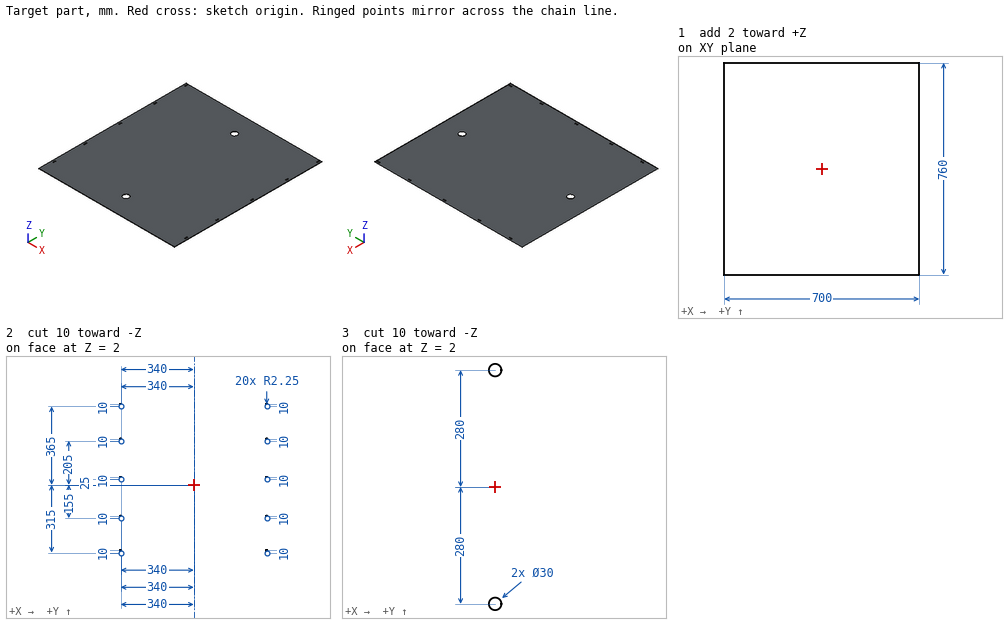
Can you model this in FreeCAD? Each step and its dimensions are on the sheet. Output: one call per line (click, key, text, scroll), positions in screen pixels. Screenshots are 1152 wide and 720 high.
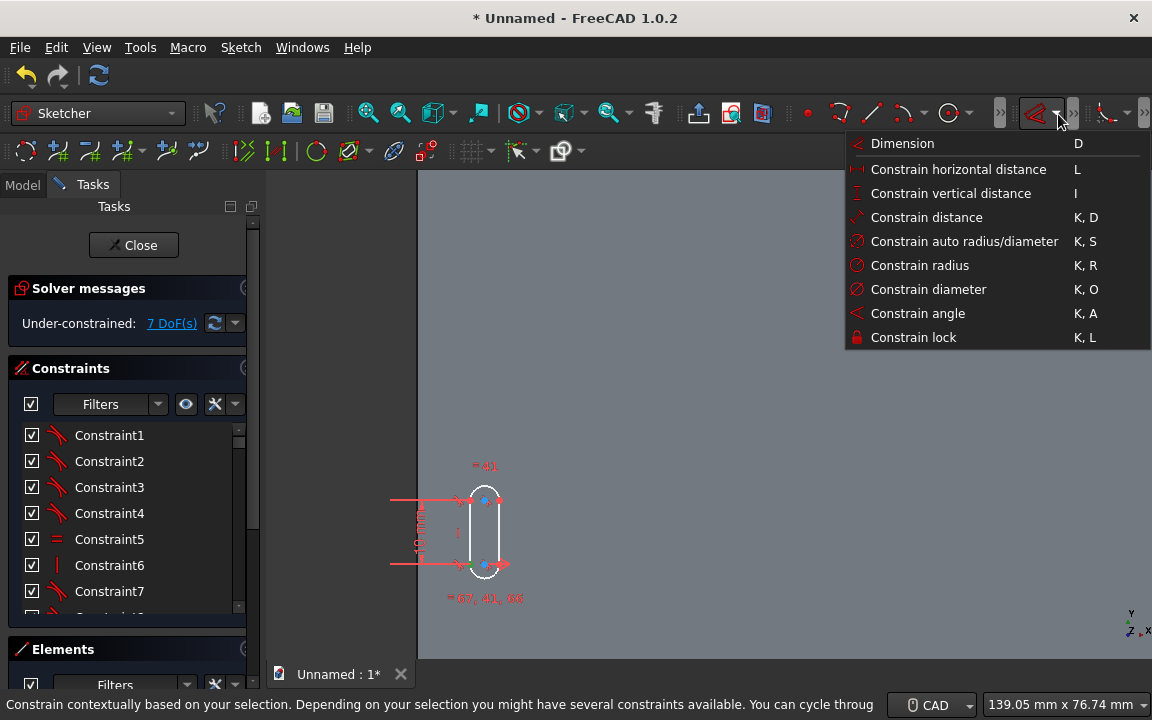
click(998, 193)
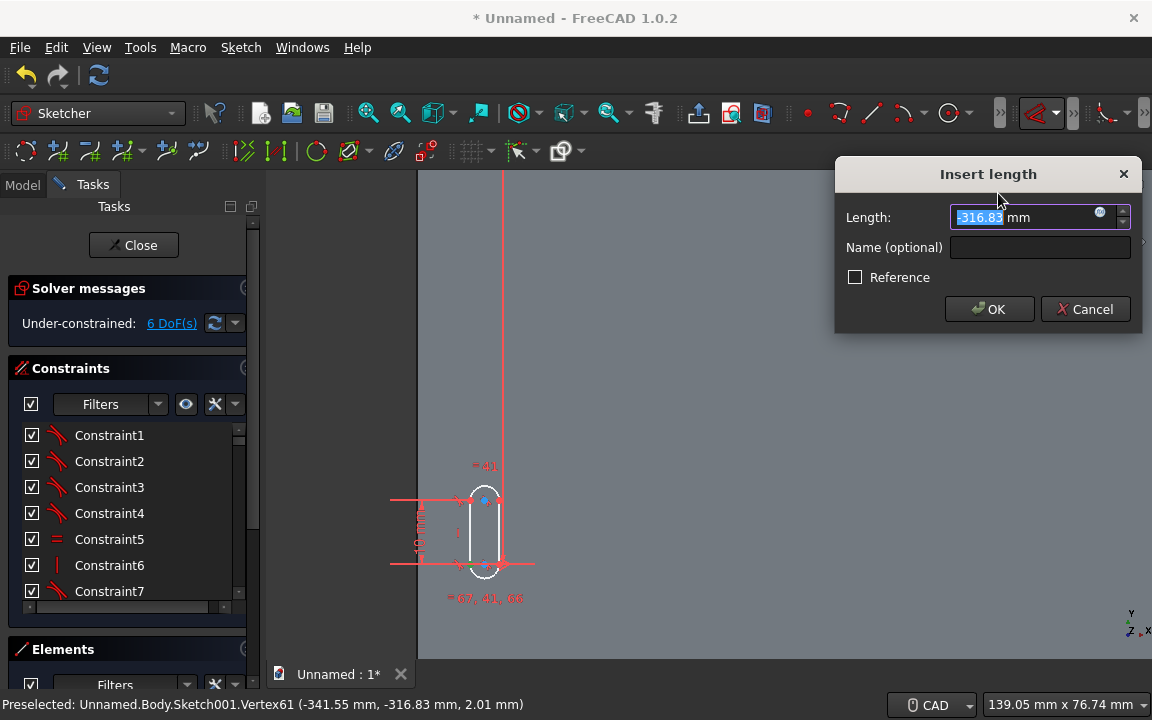
text(-315)
key(Return)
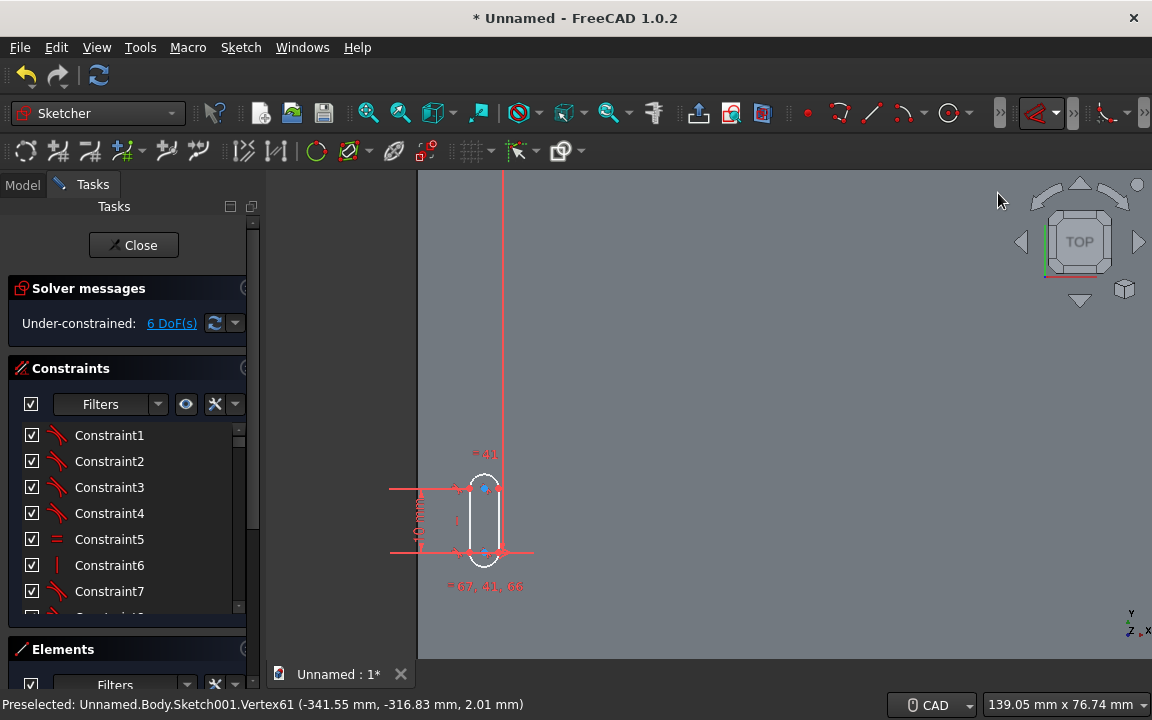
scroll(480, 580, down, 13)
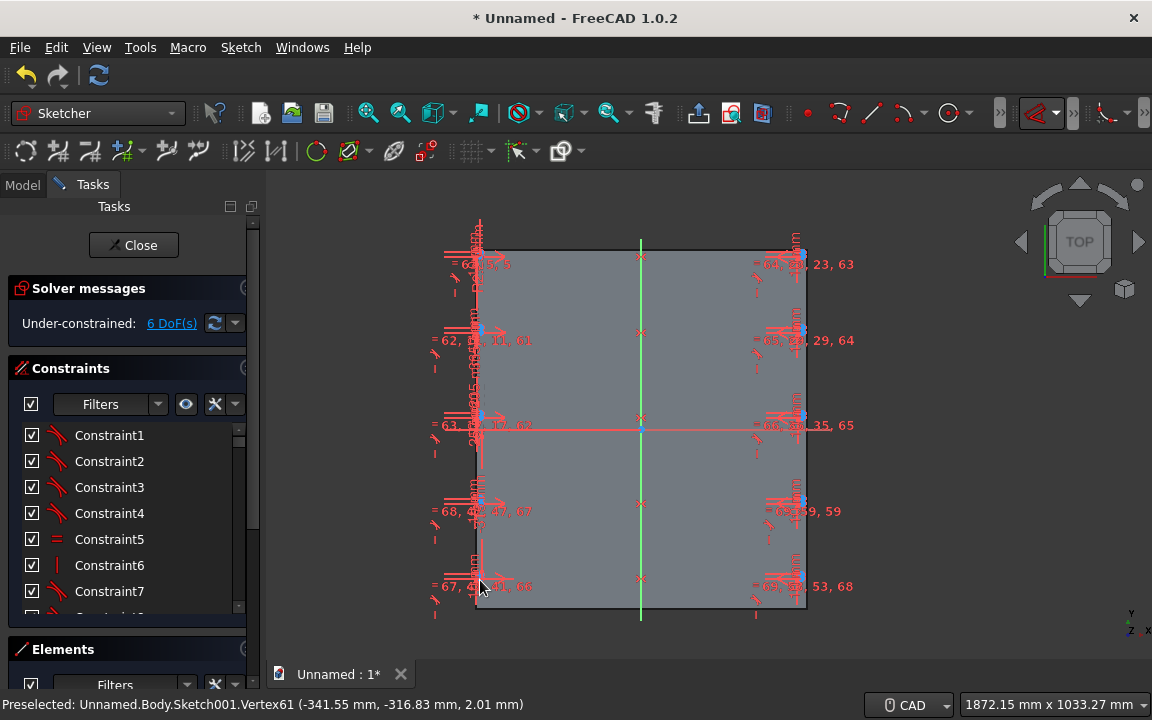
scroll(479, 504, up, 13)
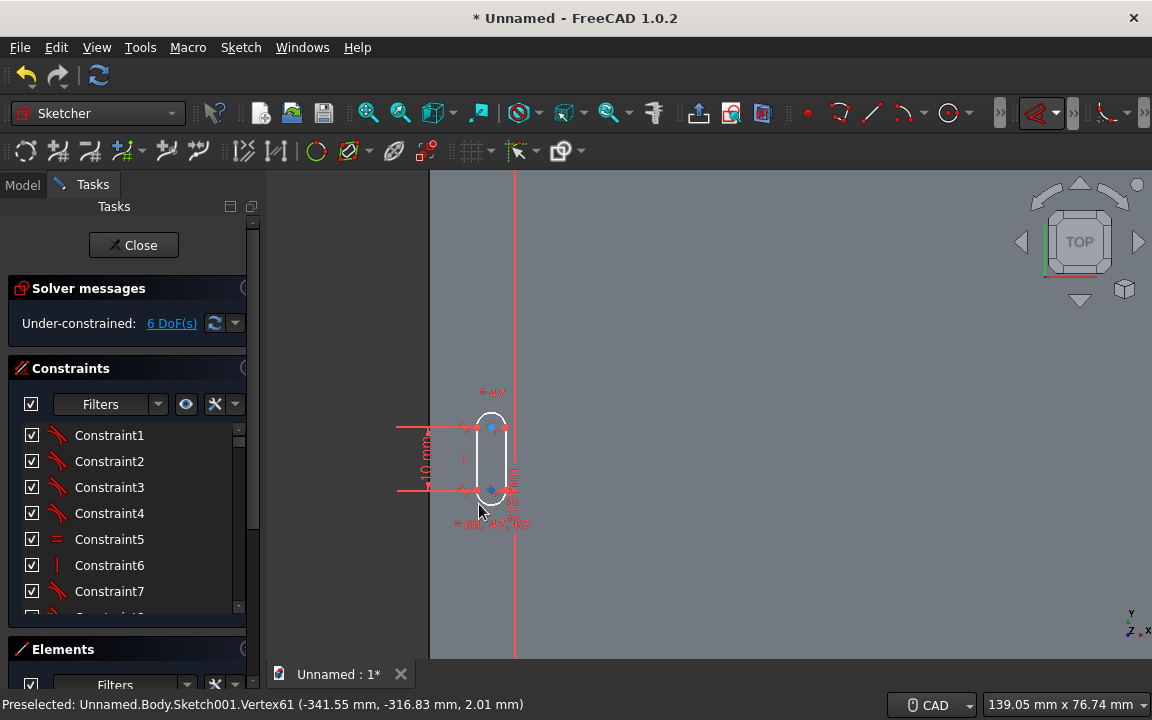
click(477, 491)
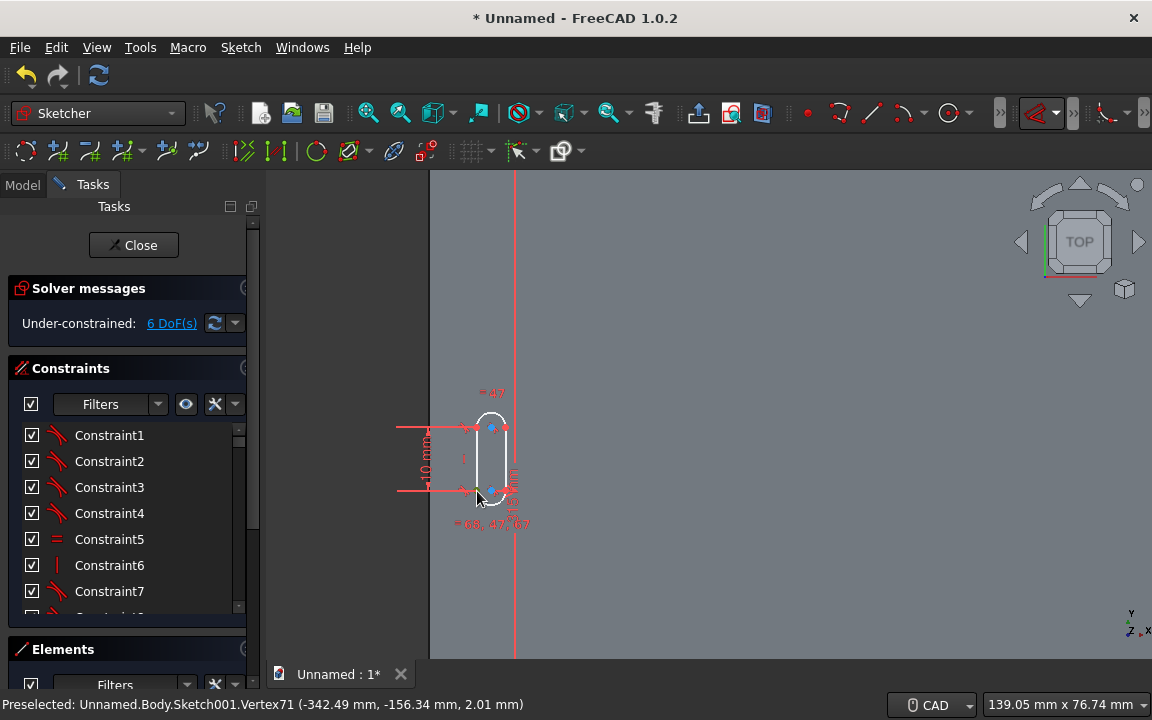
click(1058, 114)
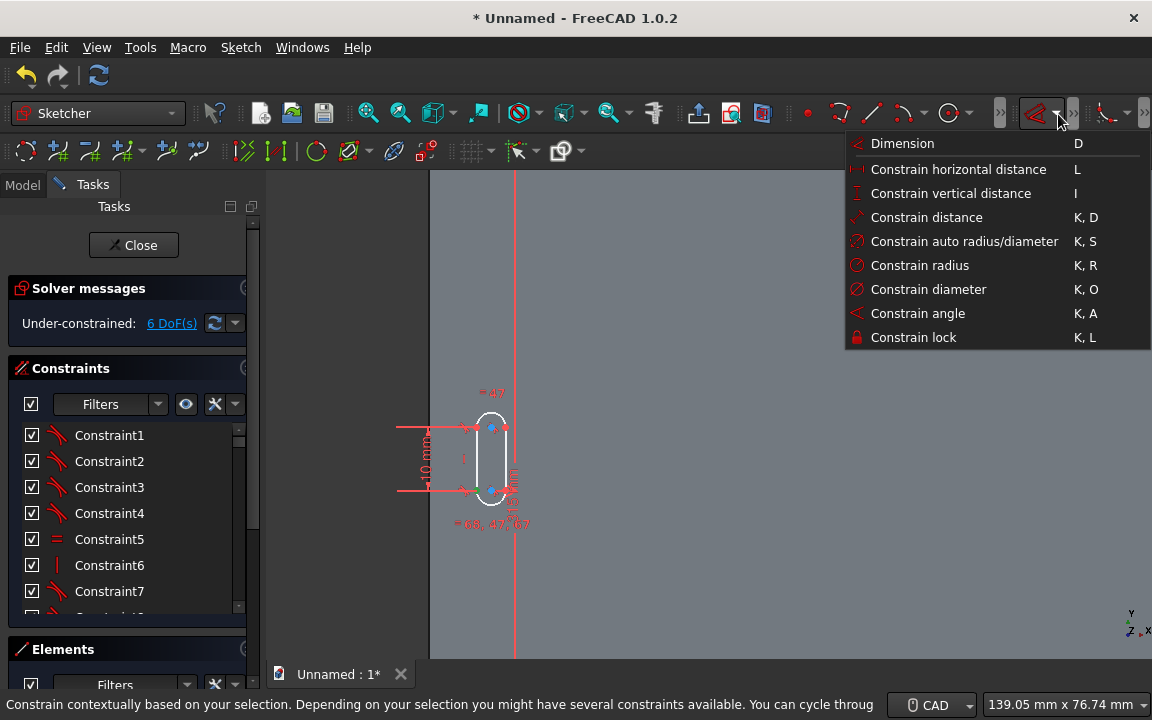
click(998, 193)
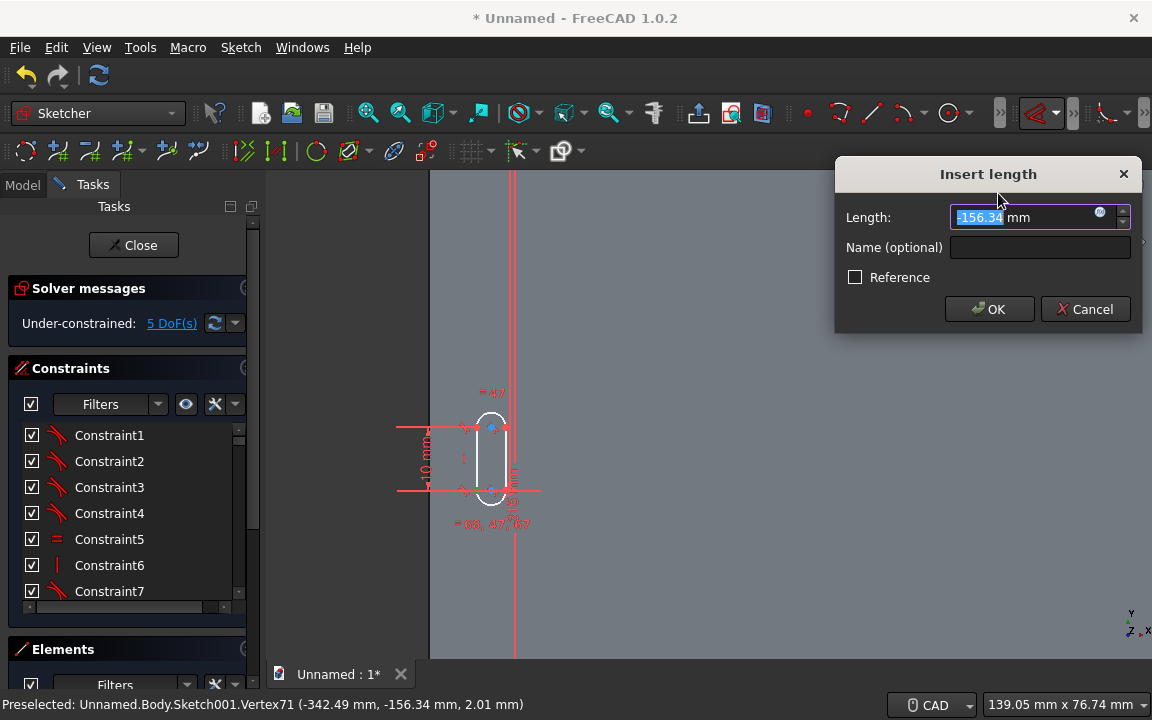
text(-155)
key(Return)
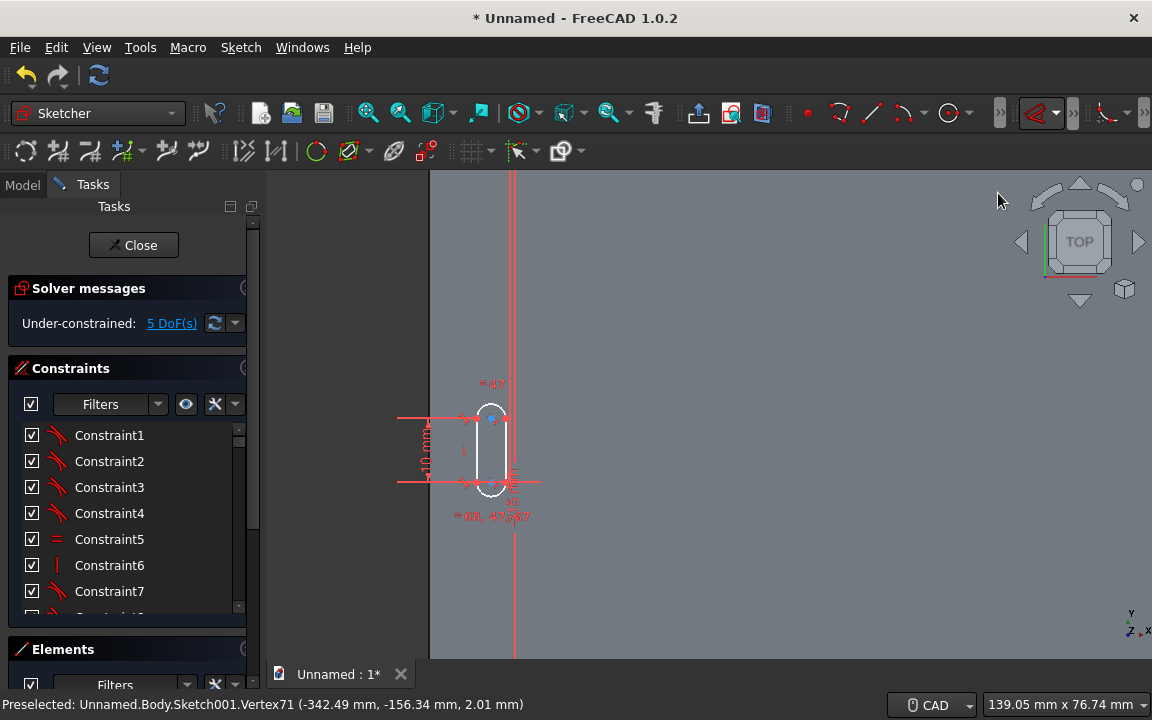
scroll(479, 504, down, 13)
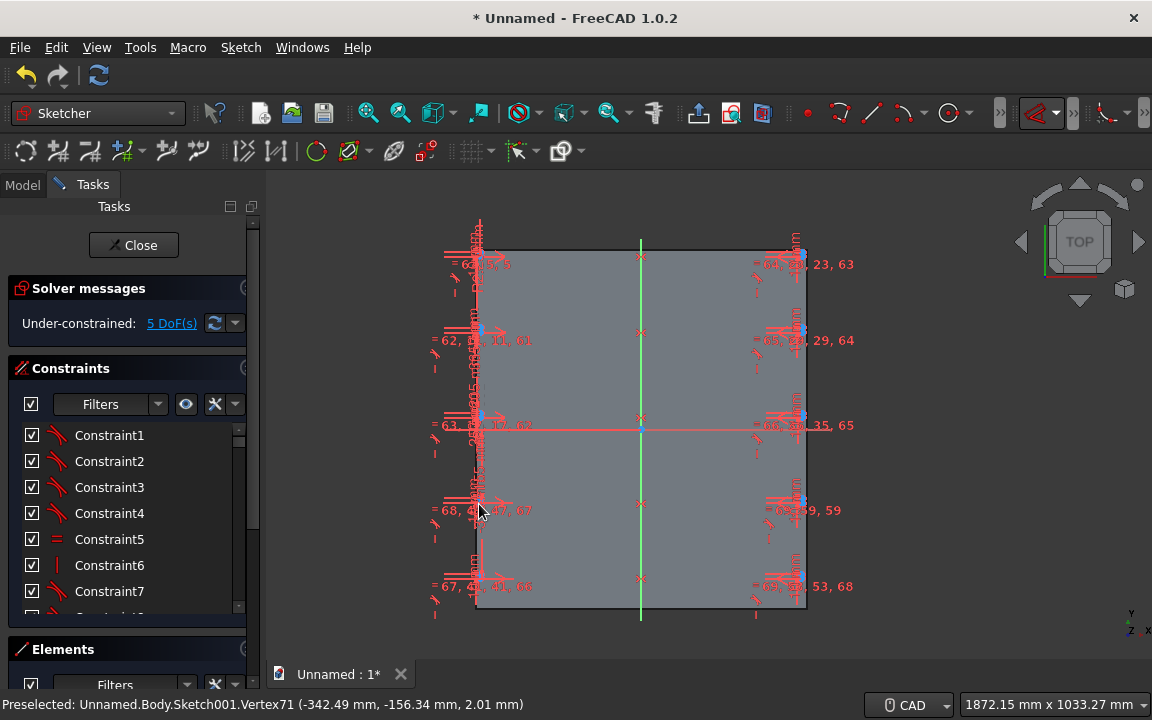
scroll(480, 257, up, 13)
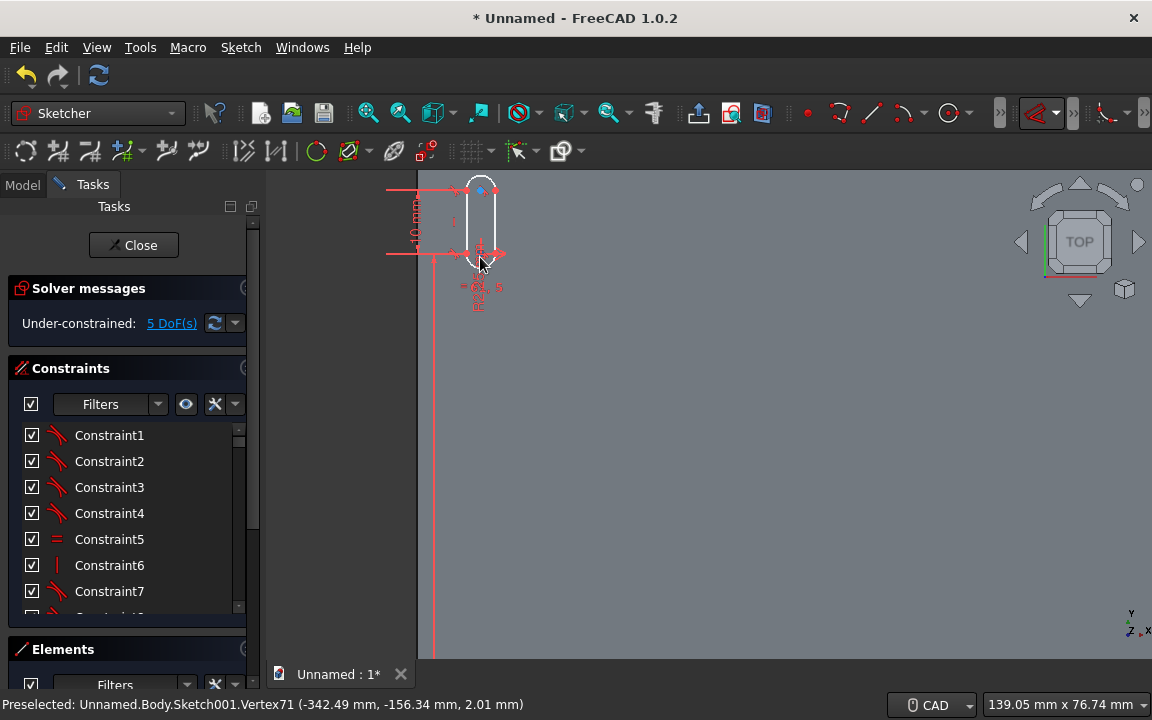
click(481, 254)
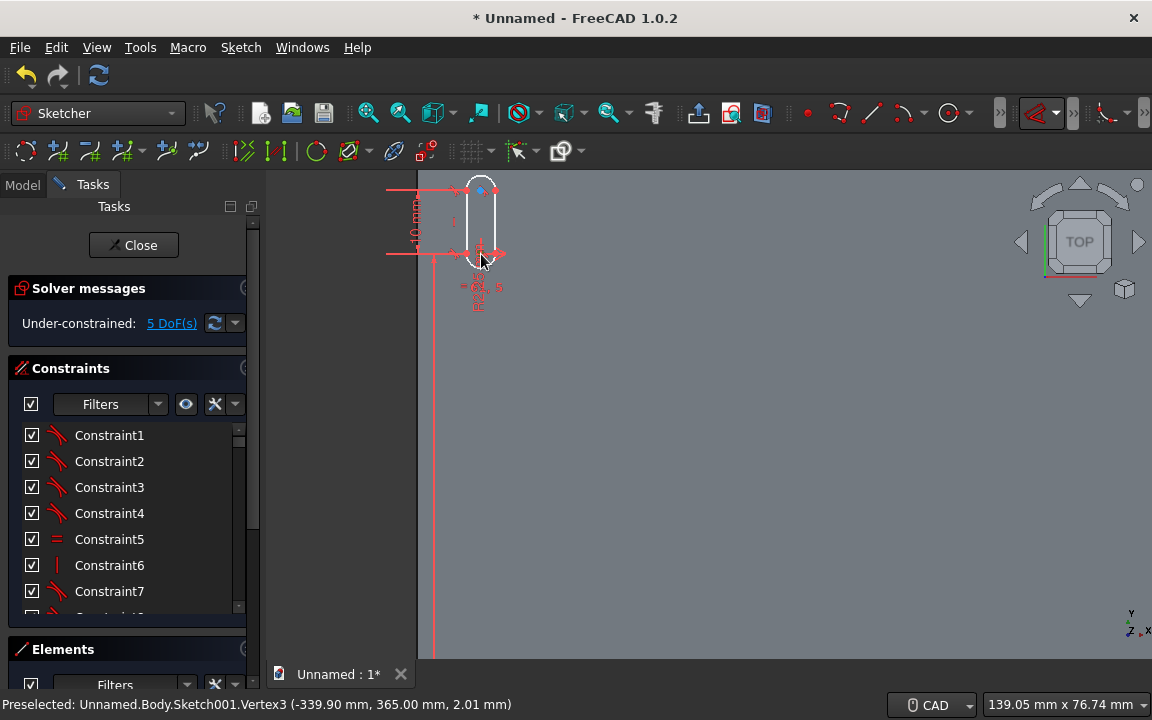
click(1058, 114)